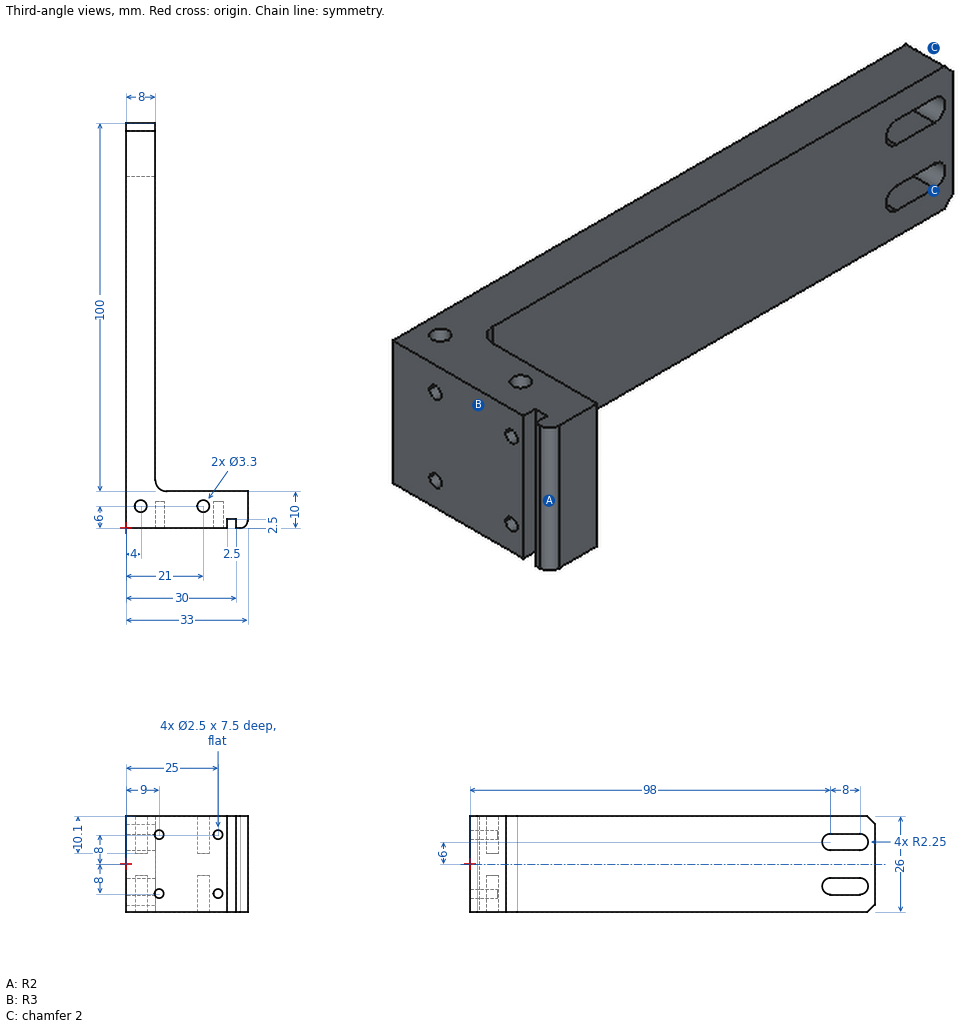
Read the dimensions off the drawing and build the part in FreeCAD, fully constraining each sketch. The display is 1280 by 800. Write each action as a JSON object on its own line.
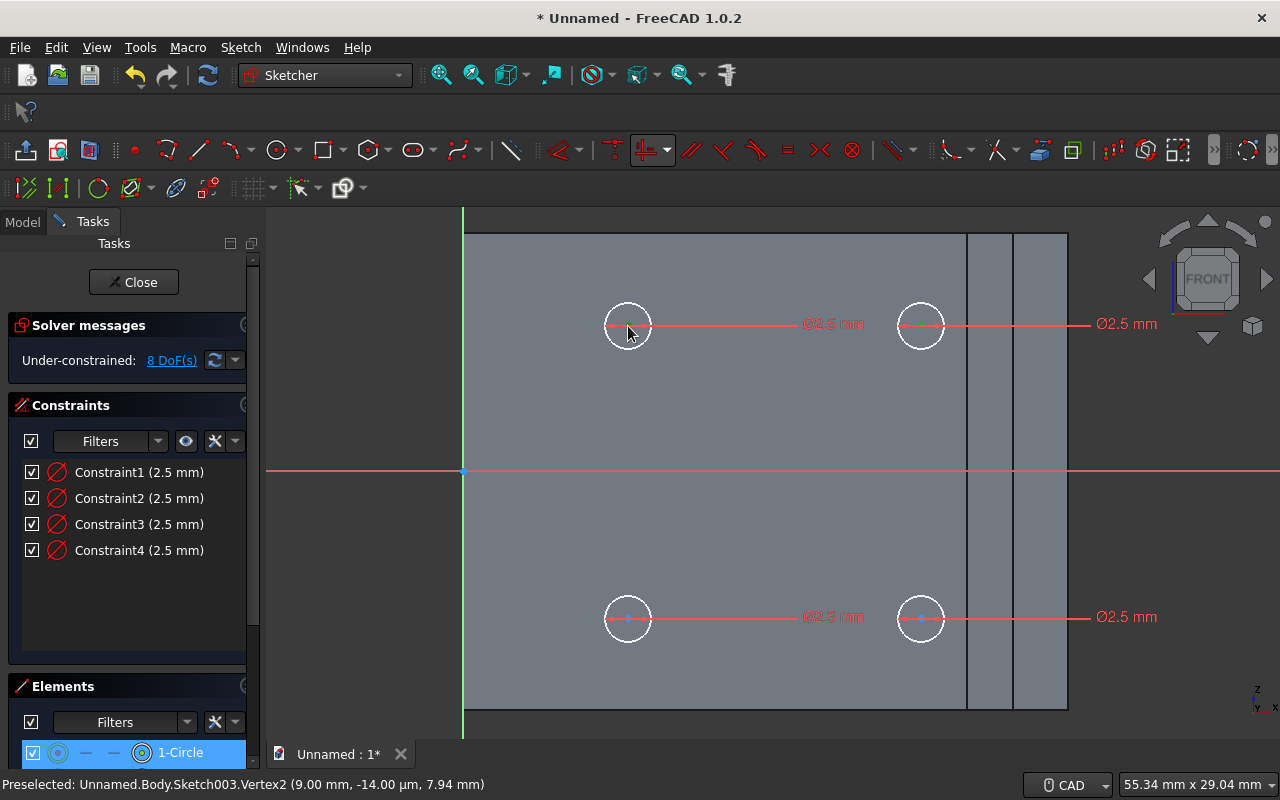
{"action": "left_click", "coordinate": [670, 150]}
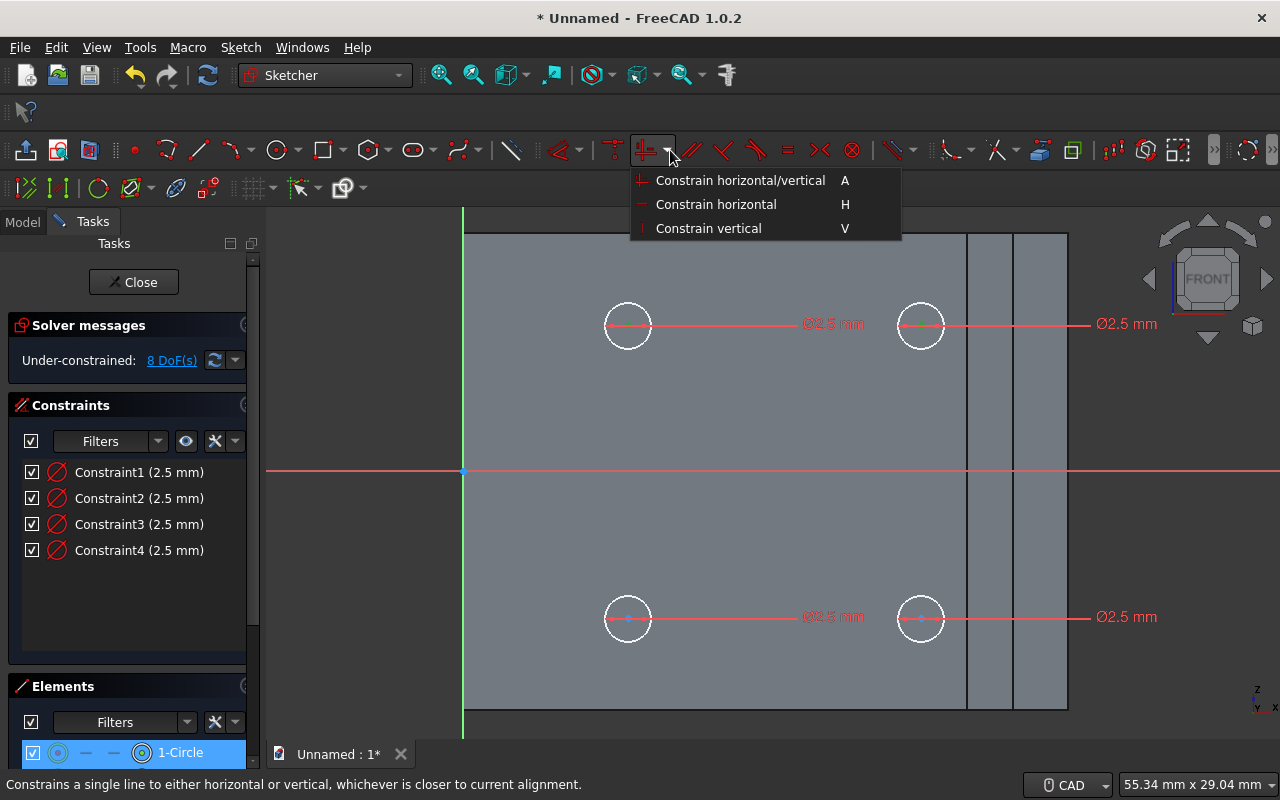
{"action": "left_click", "coordinate": [766, 204]}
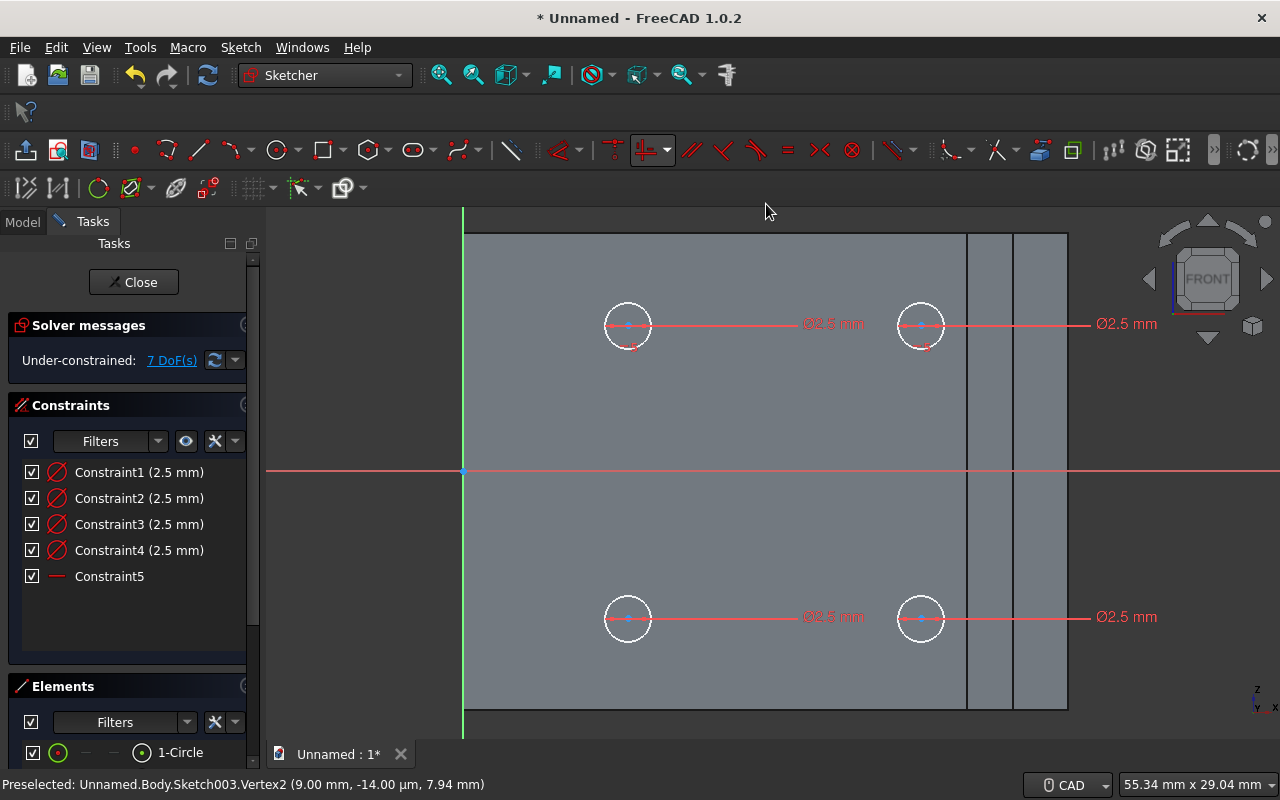
{"action": "left_click", "coordinate": [628, 326]}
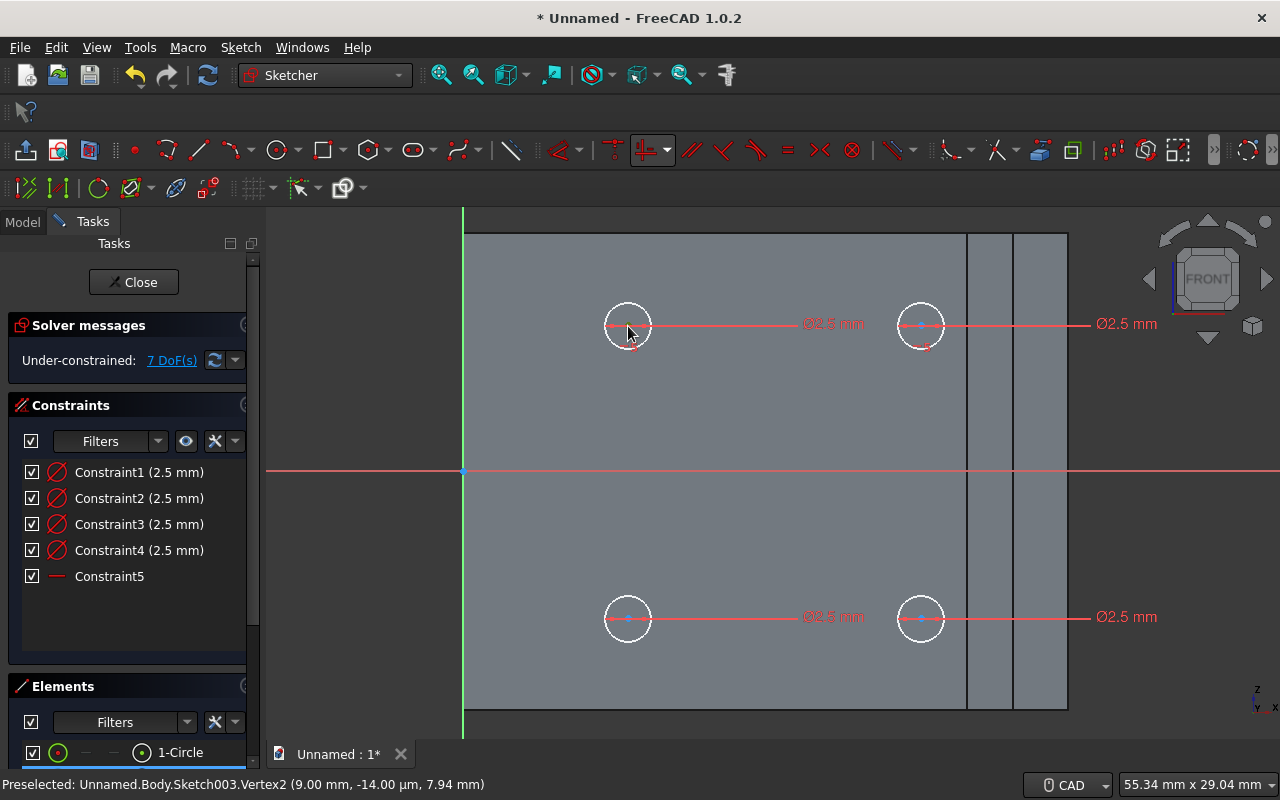
{"action": "left_click", "coordinate": [628, 619]}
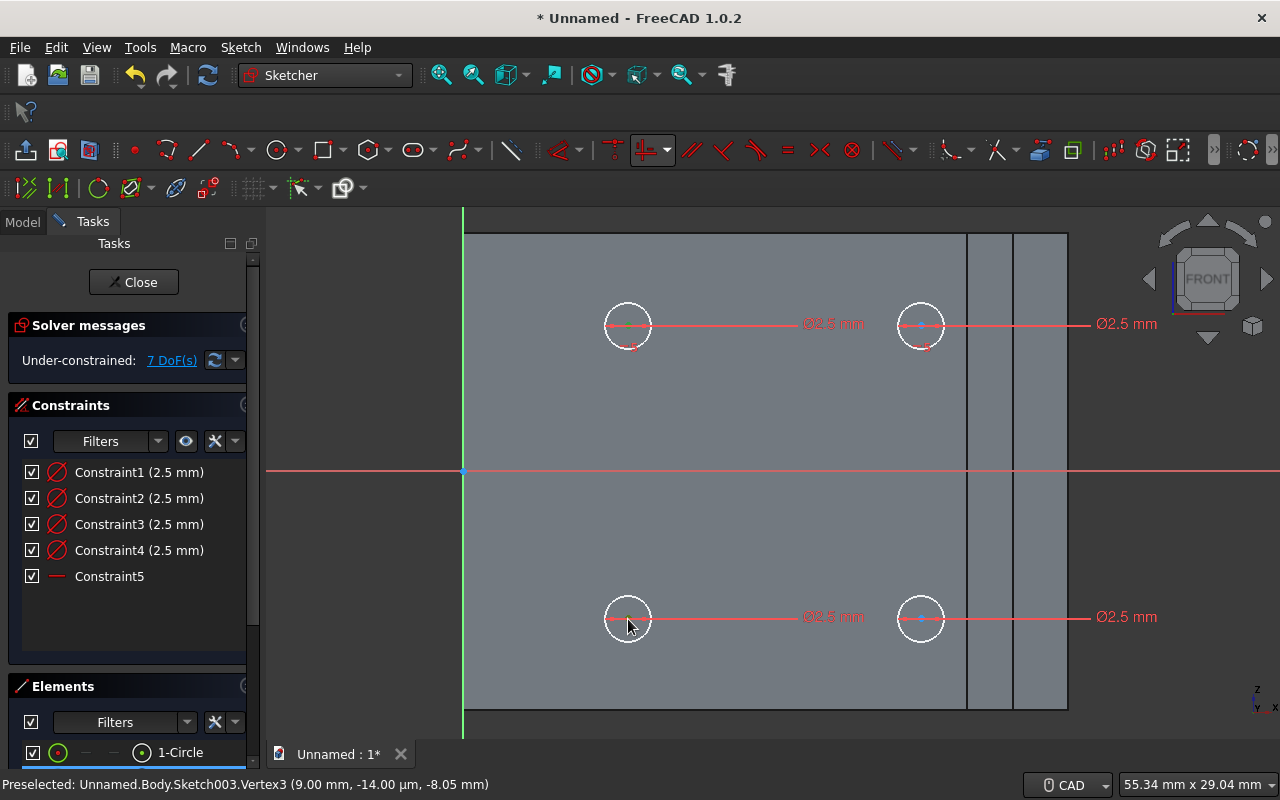
{"action": "key", "text": "v"}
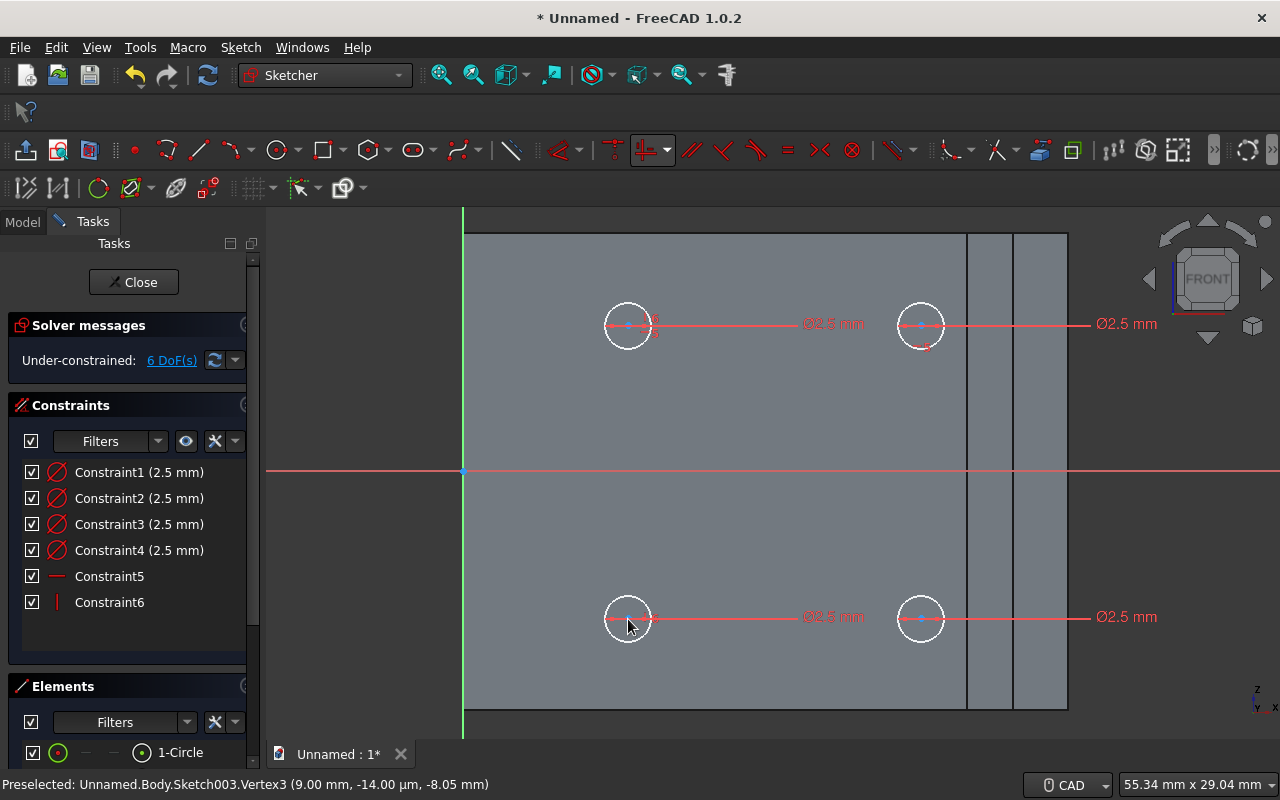
{"action": "left_click", "coordinate": [921, 326]}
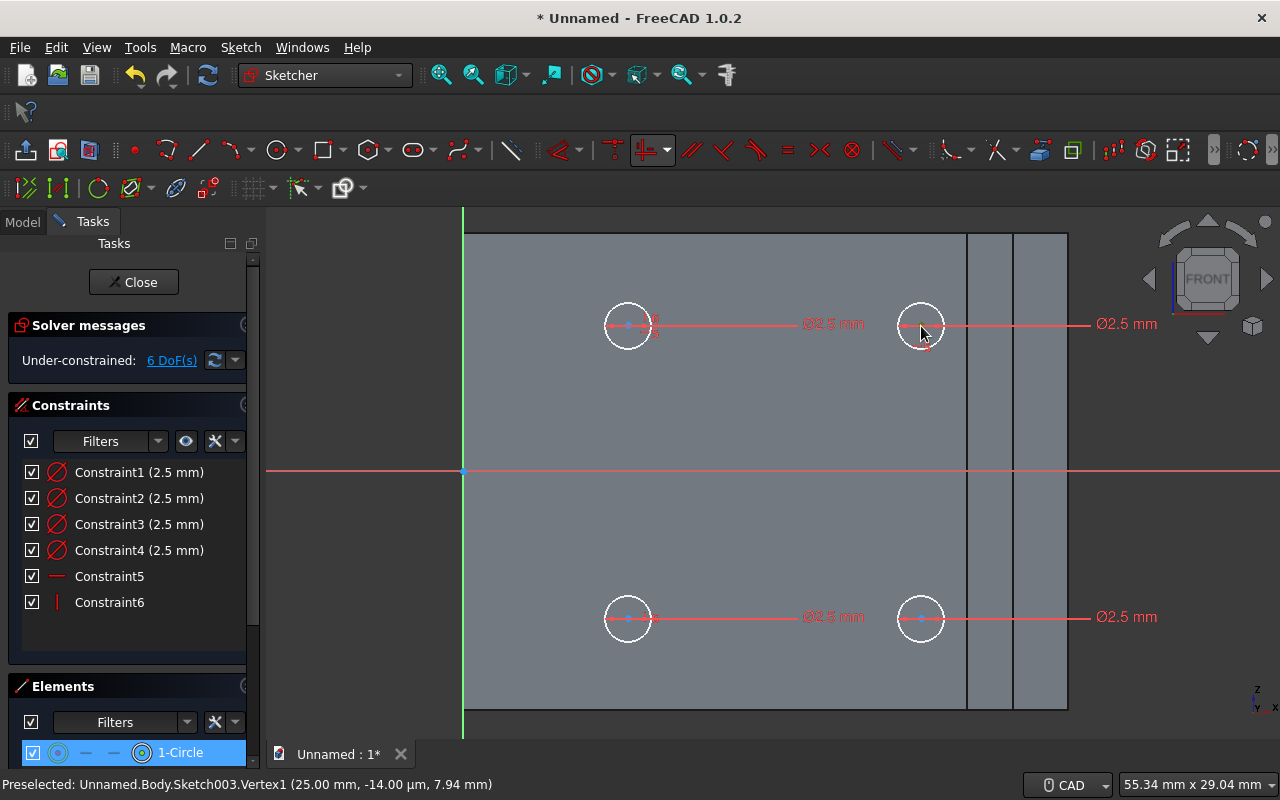
{"action": "left_click", "coordinate": [921, 619]}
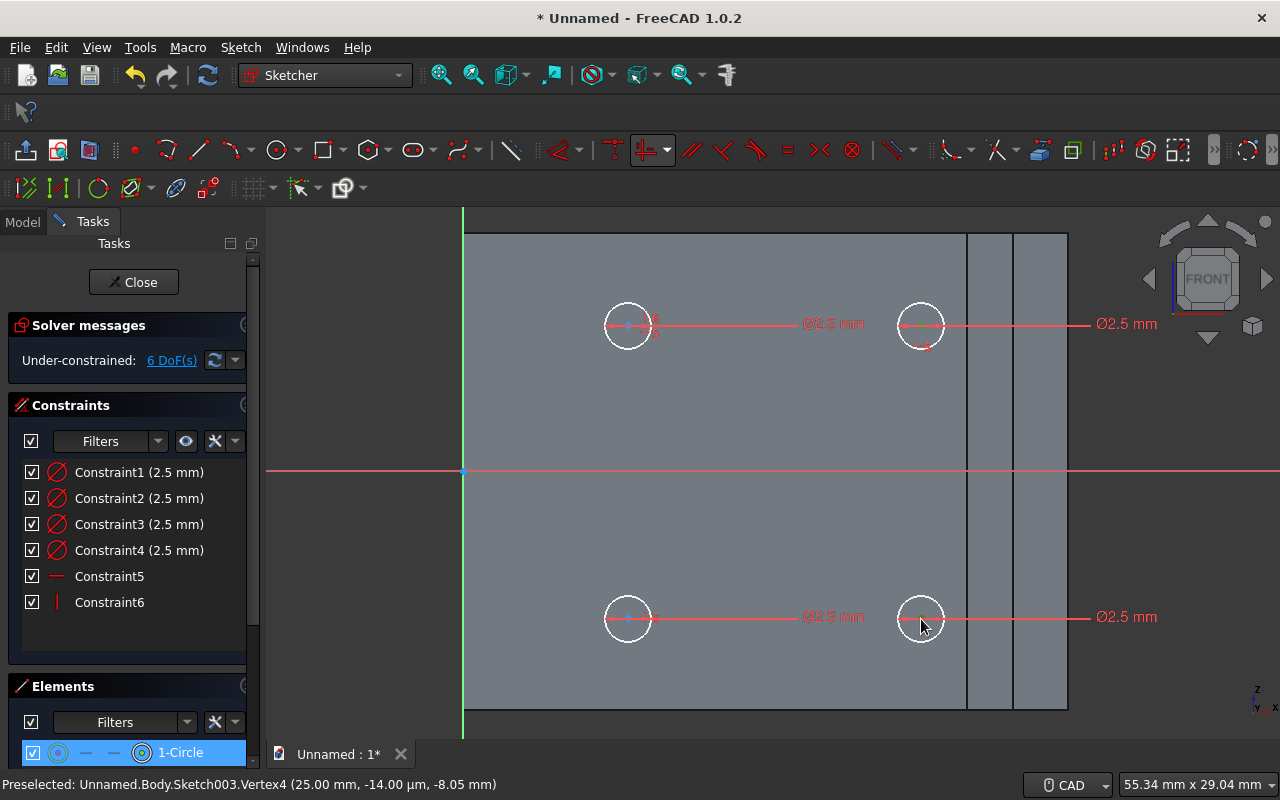
{"action": "key", "text": "v"}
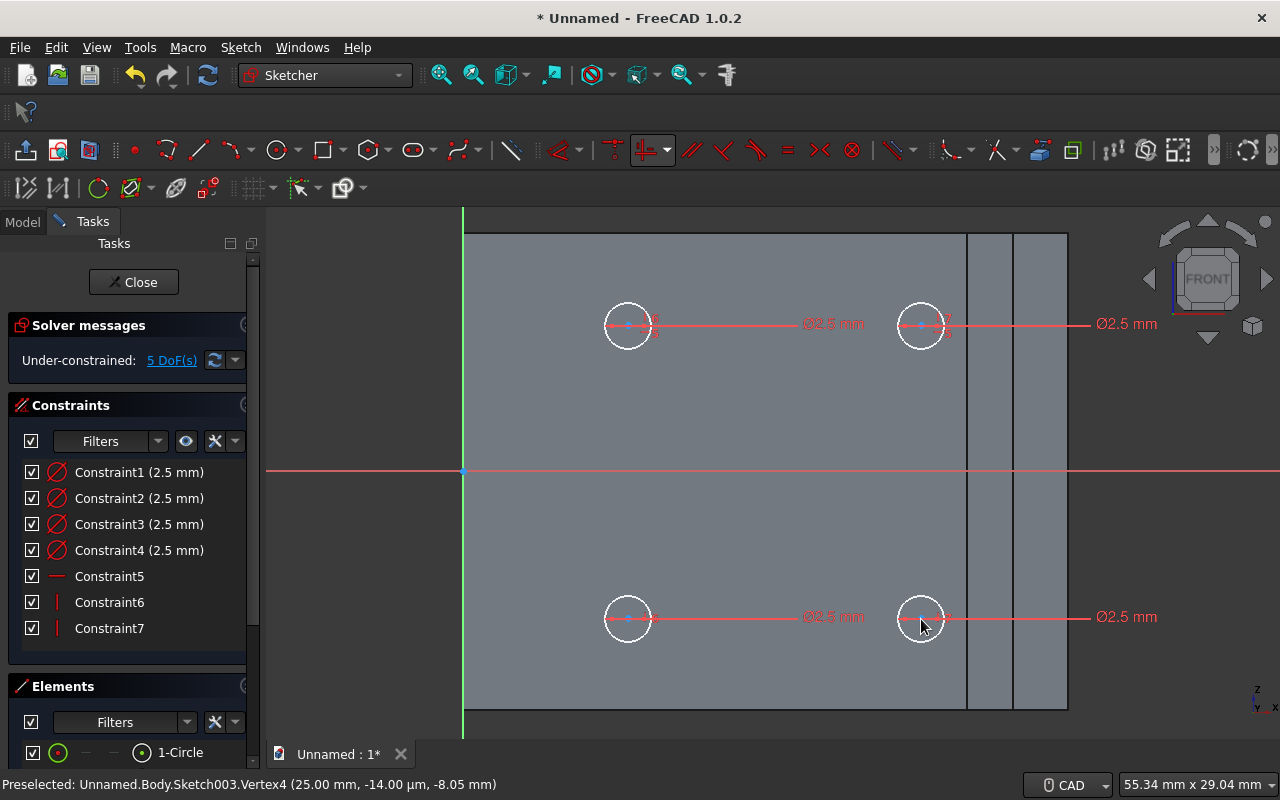
{"action": "left_click", "coordinate": [628, 619]}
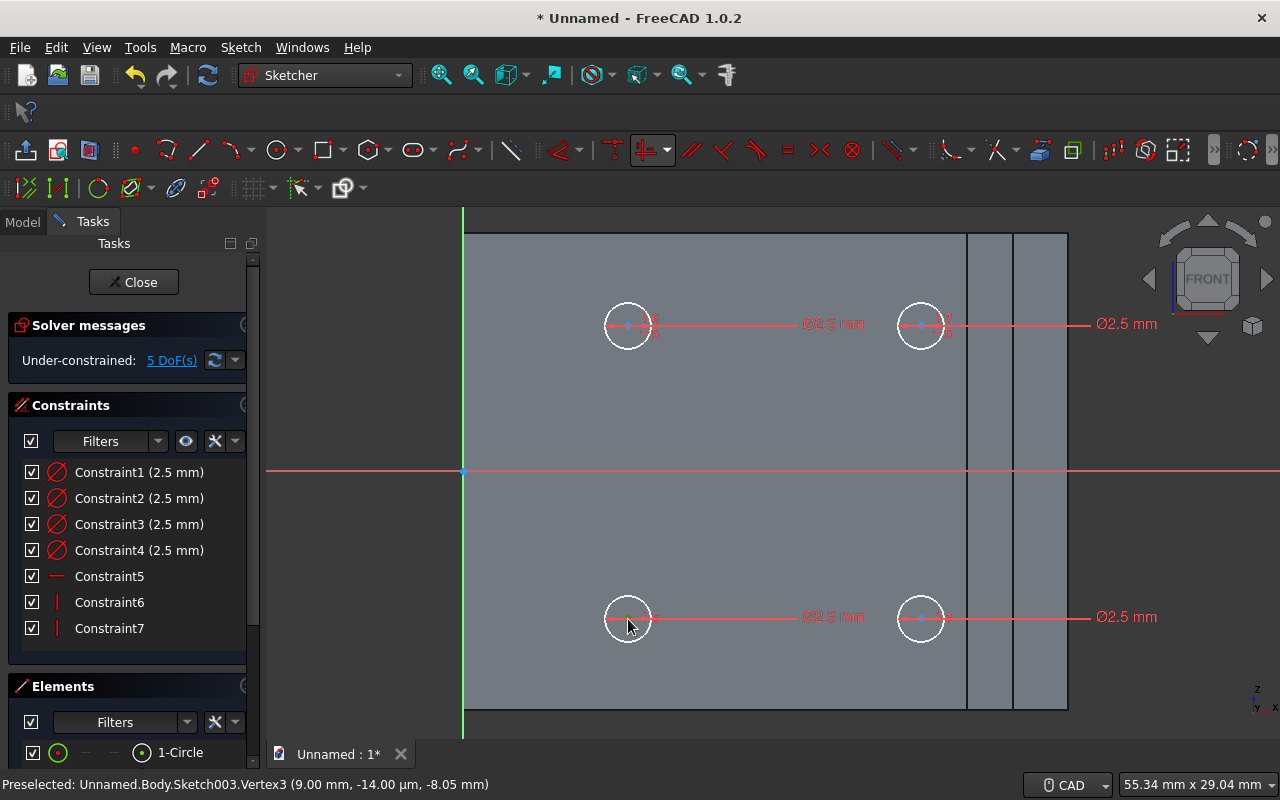
{"action": "left_click", "coordinate": [921, 619]}